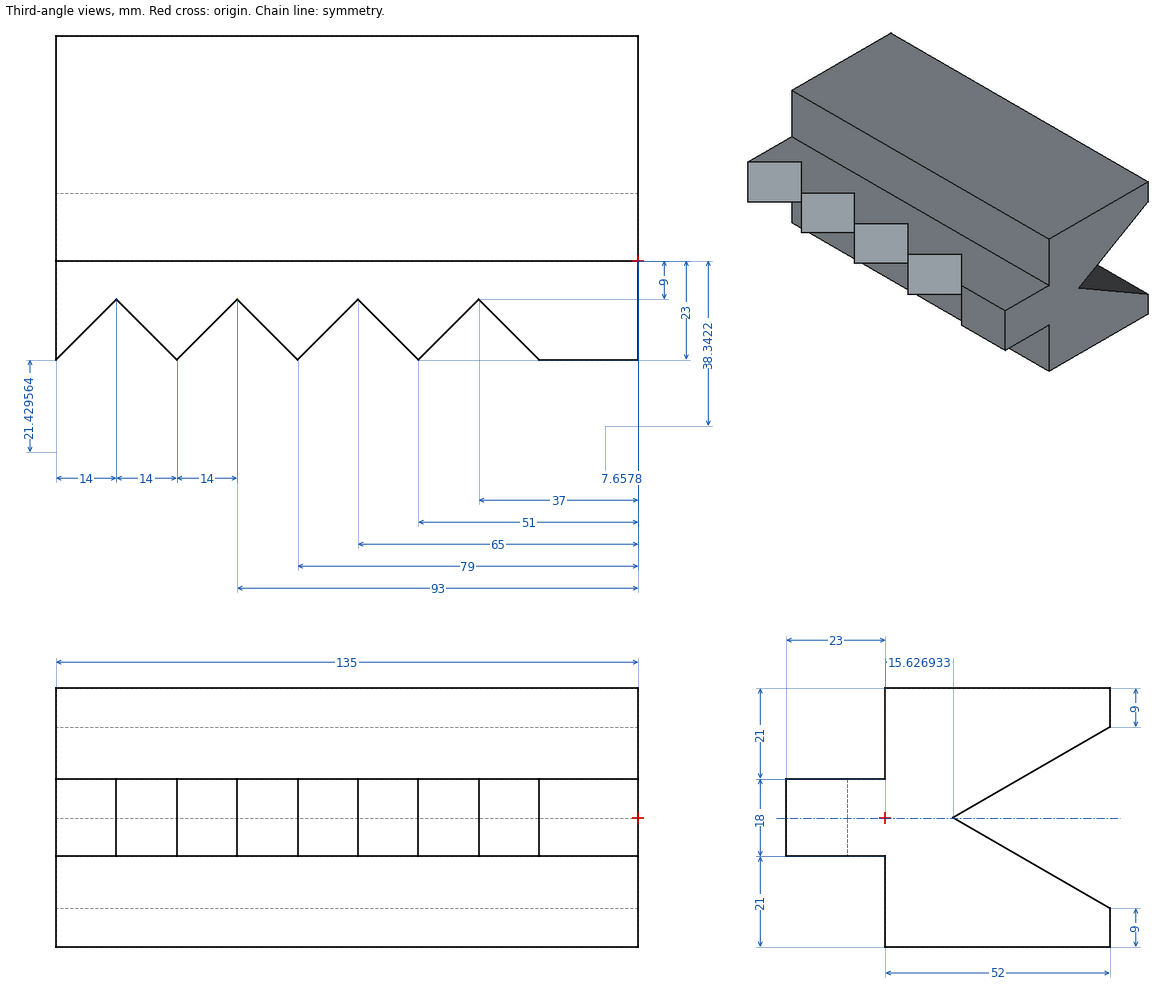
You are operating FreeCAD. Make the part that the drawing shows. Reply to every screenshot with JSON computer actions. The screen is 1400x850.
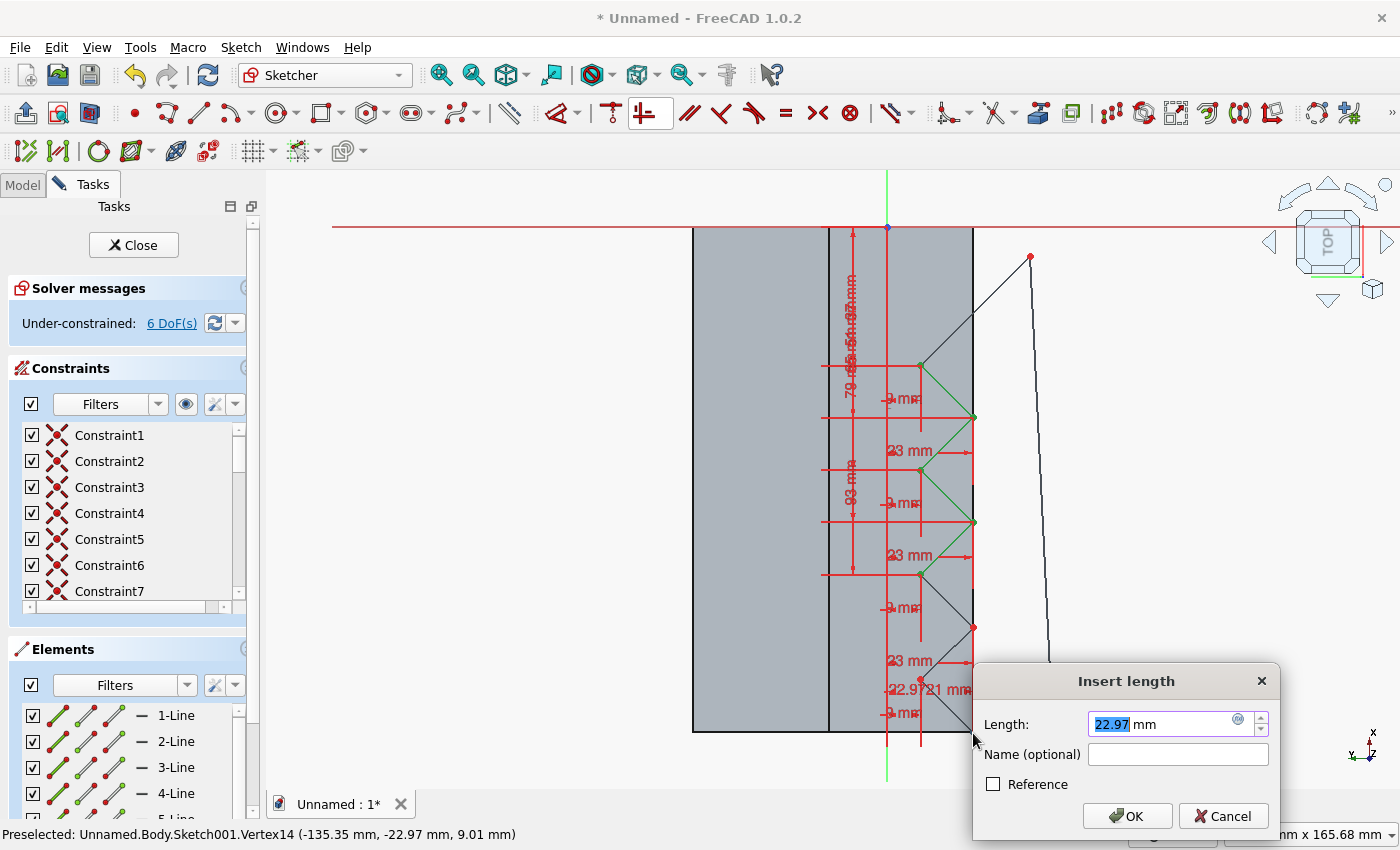
{"action": "type", "text": "23"}
{"action": "key", "text": "Return"}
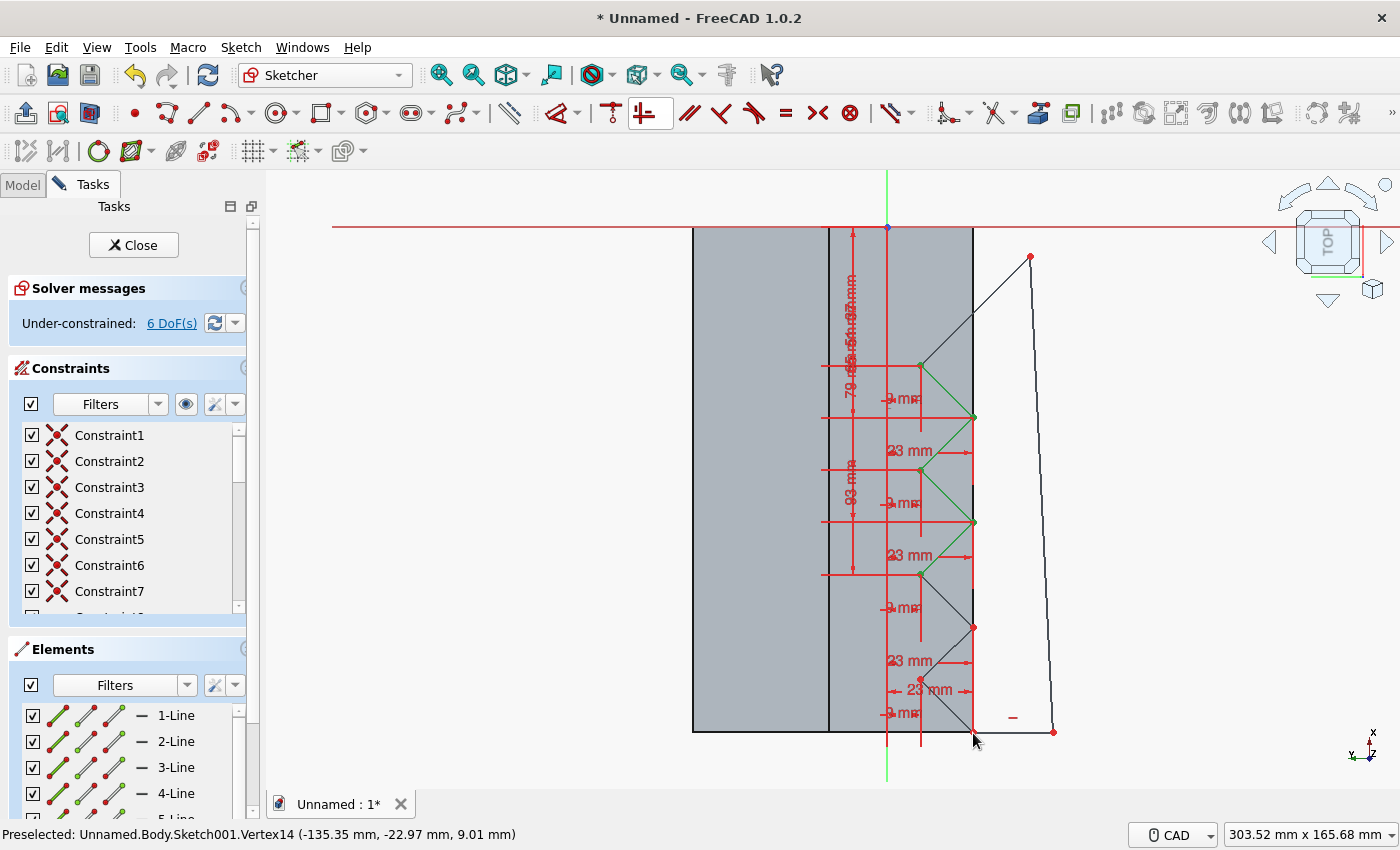
{"action": "left_click", "coordinate": [936, 591]}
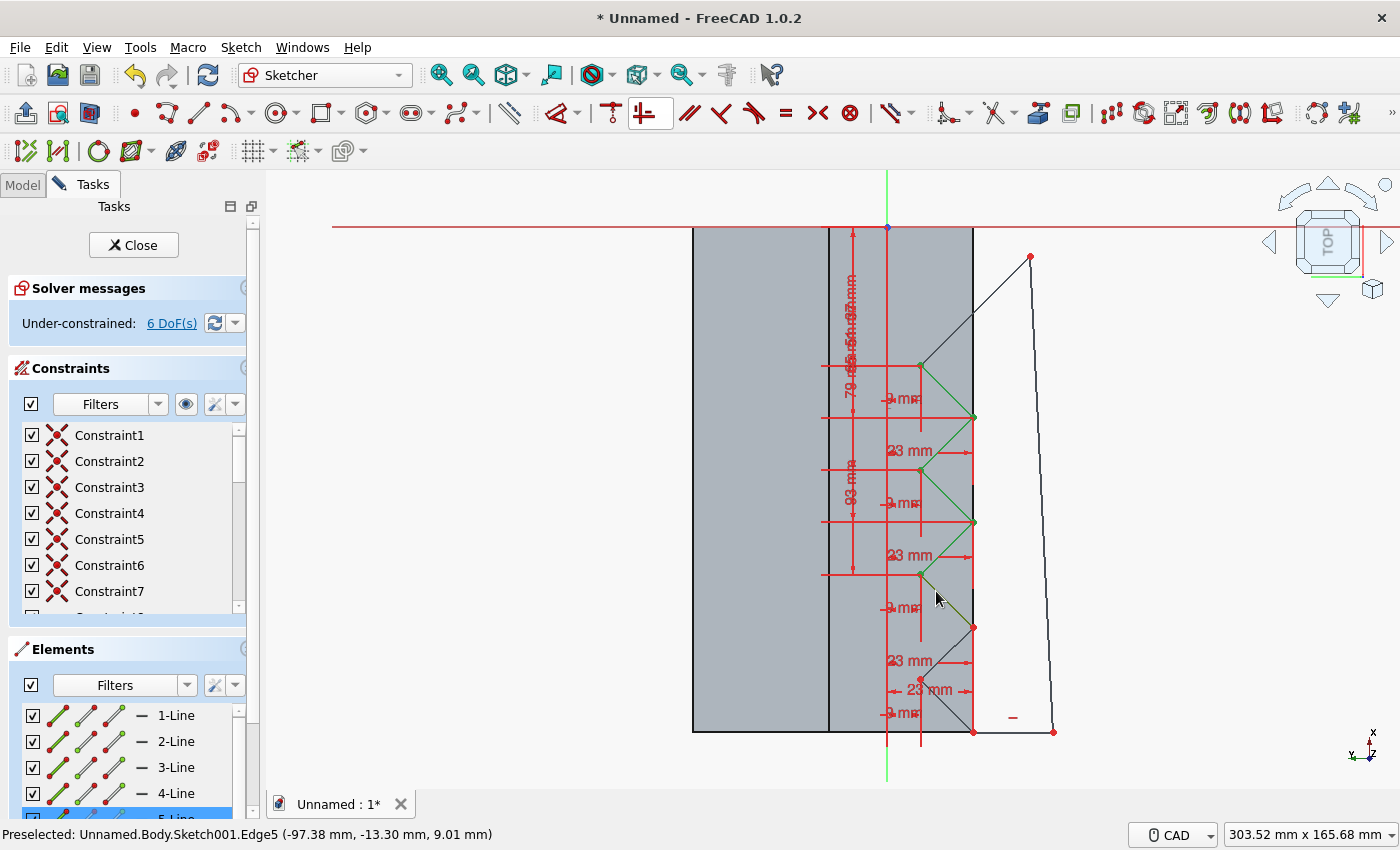
{"action": "left_click", "coordinate": [580, 114]}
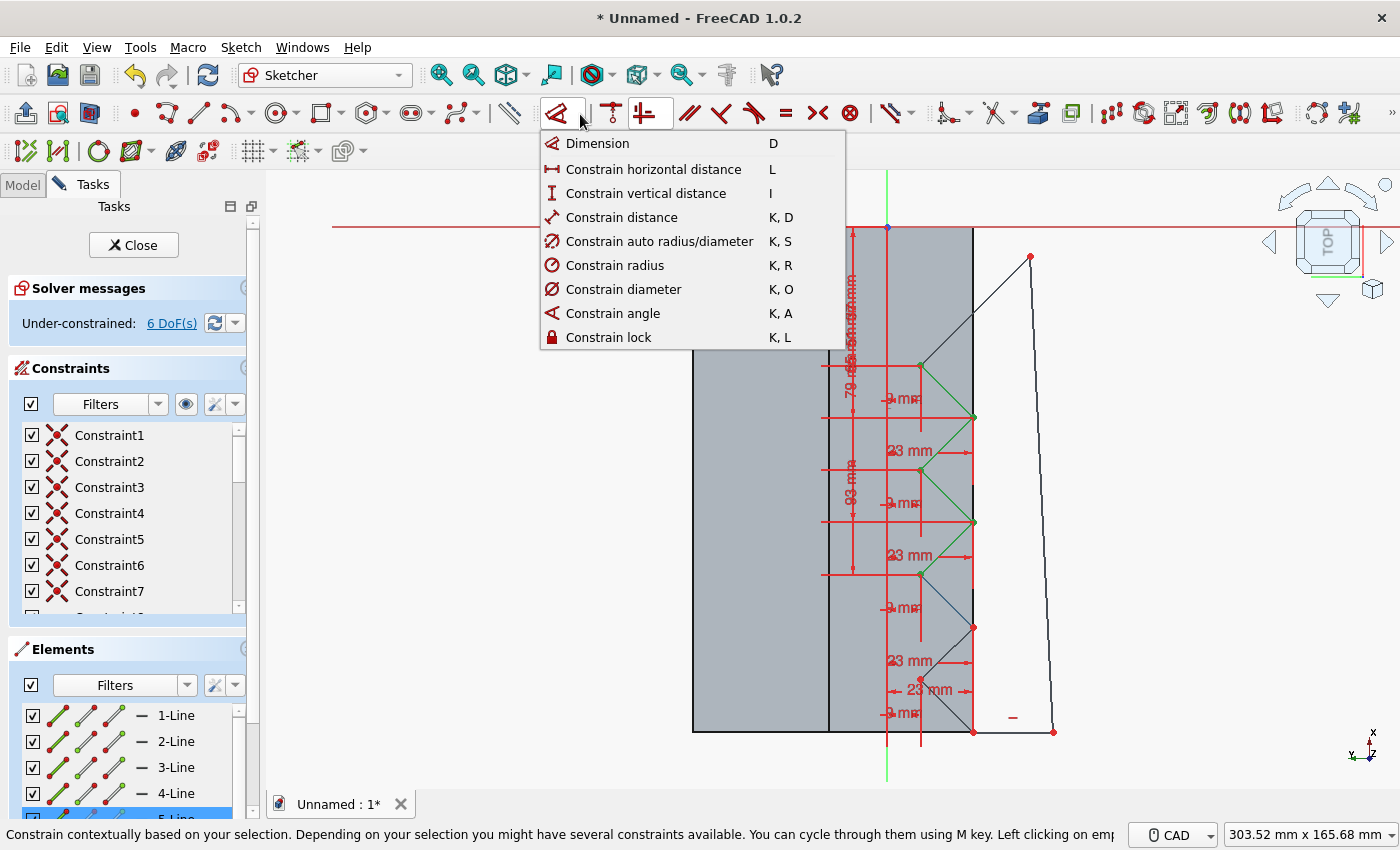
{"action": "left_click", "coordinate": [693, 193]}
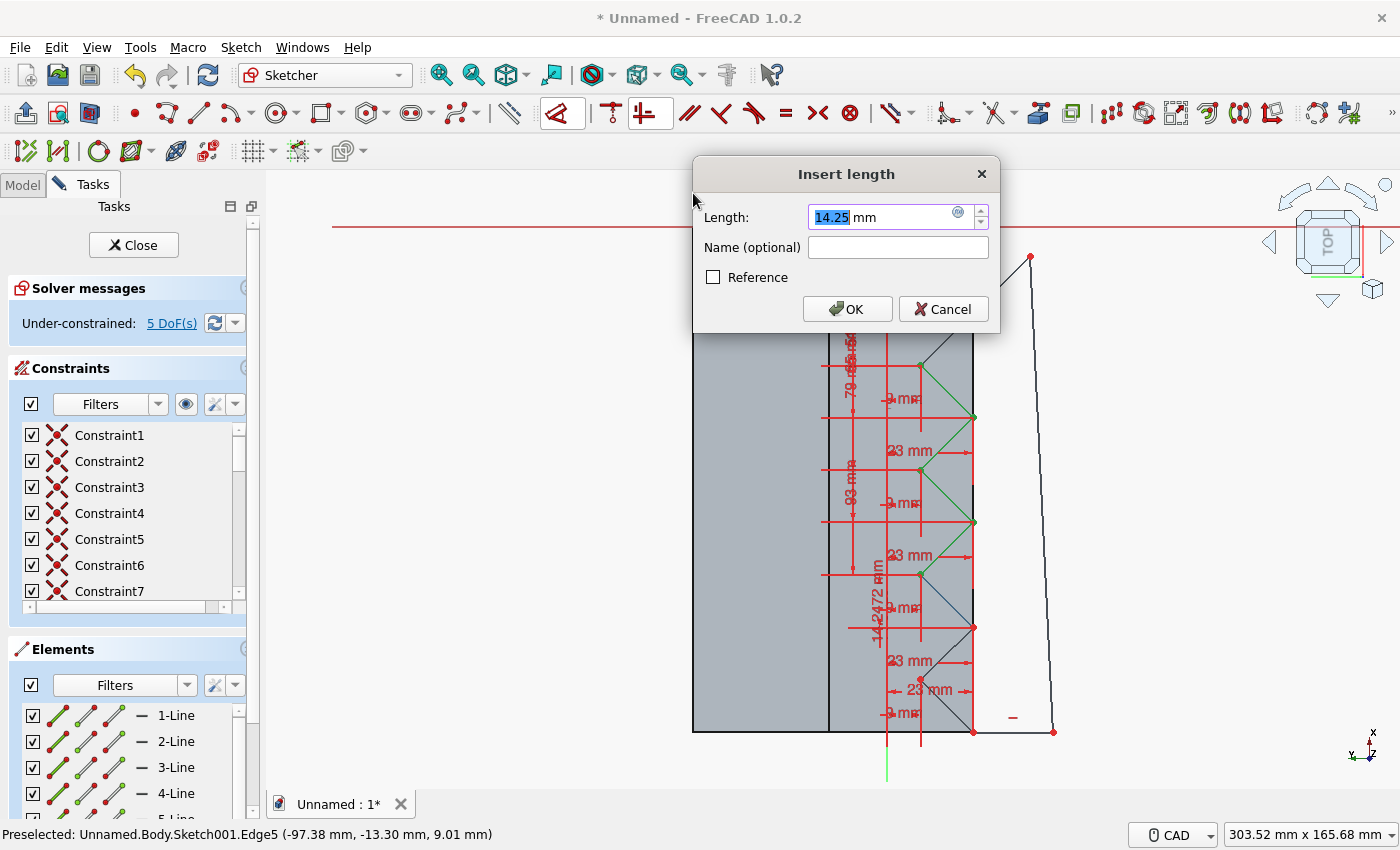
{"action": "type", "text": "14"}
{"action": "key", "text": "Return"}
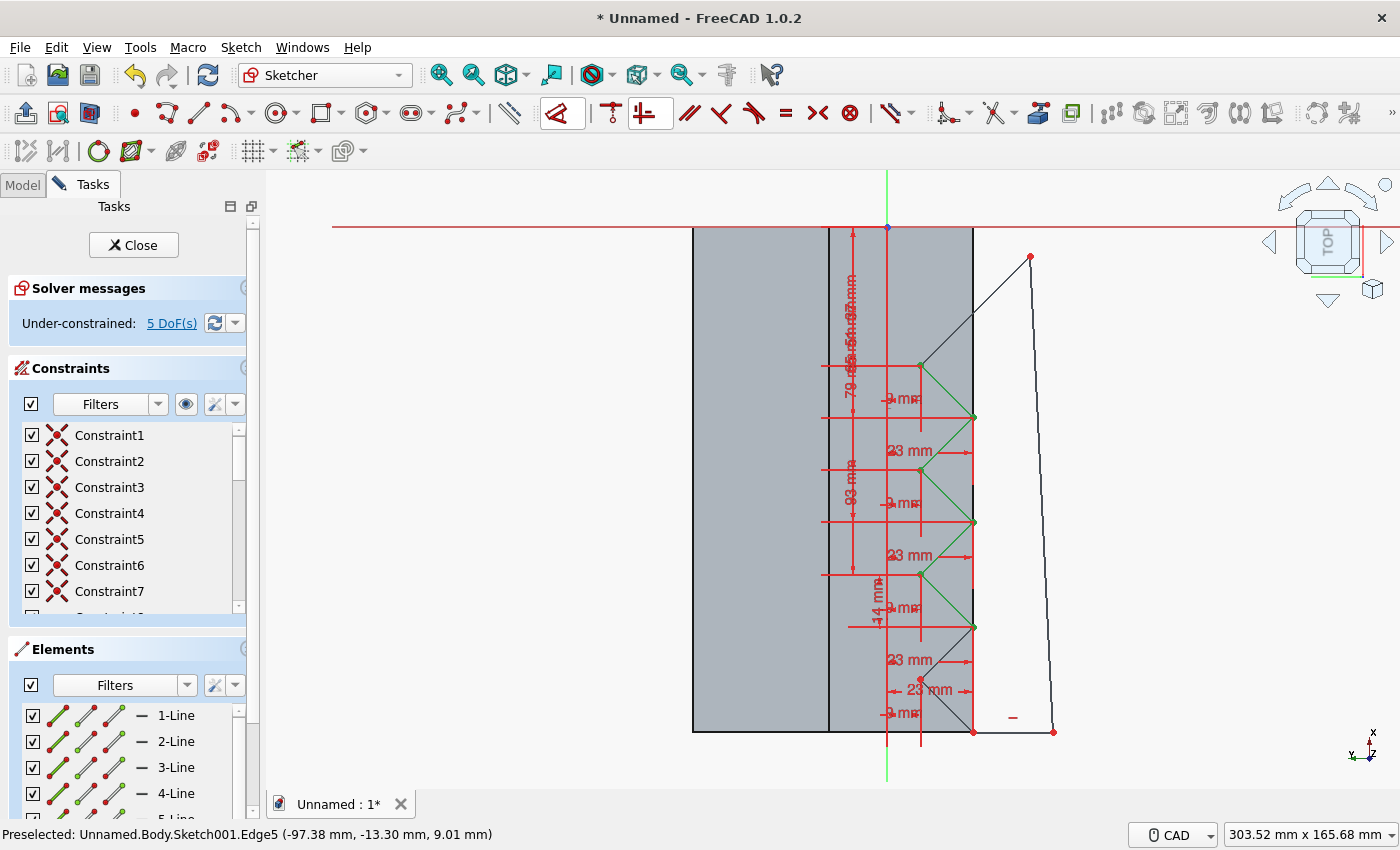
{"action": "left_click", "coordinate": [957, 643]}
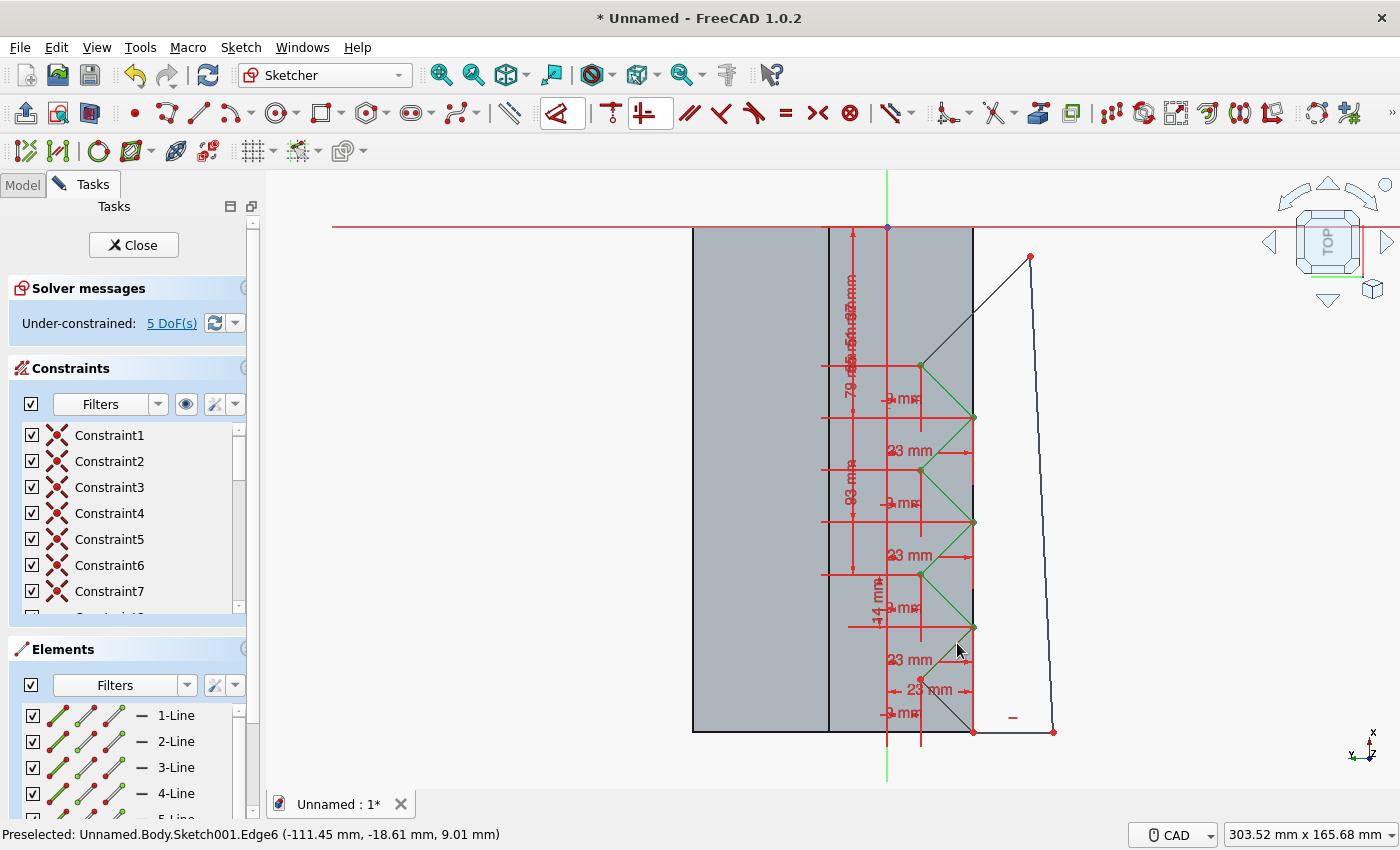
{"action": "key", "text": "i"}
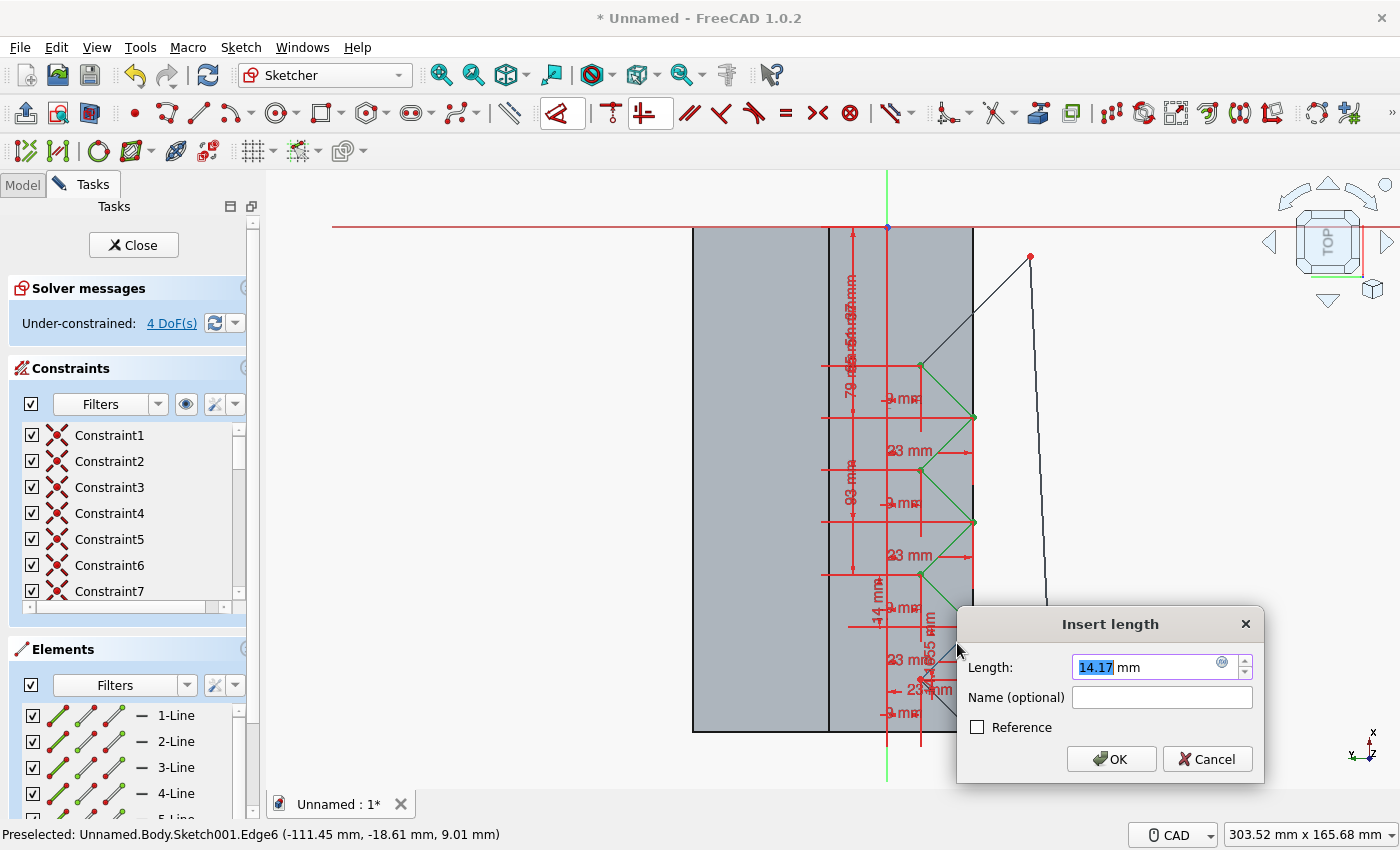
{"action": "type", "text": "14"}
{"action": "key", "text": "Return"}